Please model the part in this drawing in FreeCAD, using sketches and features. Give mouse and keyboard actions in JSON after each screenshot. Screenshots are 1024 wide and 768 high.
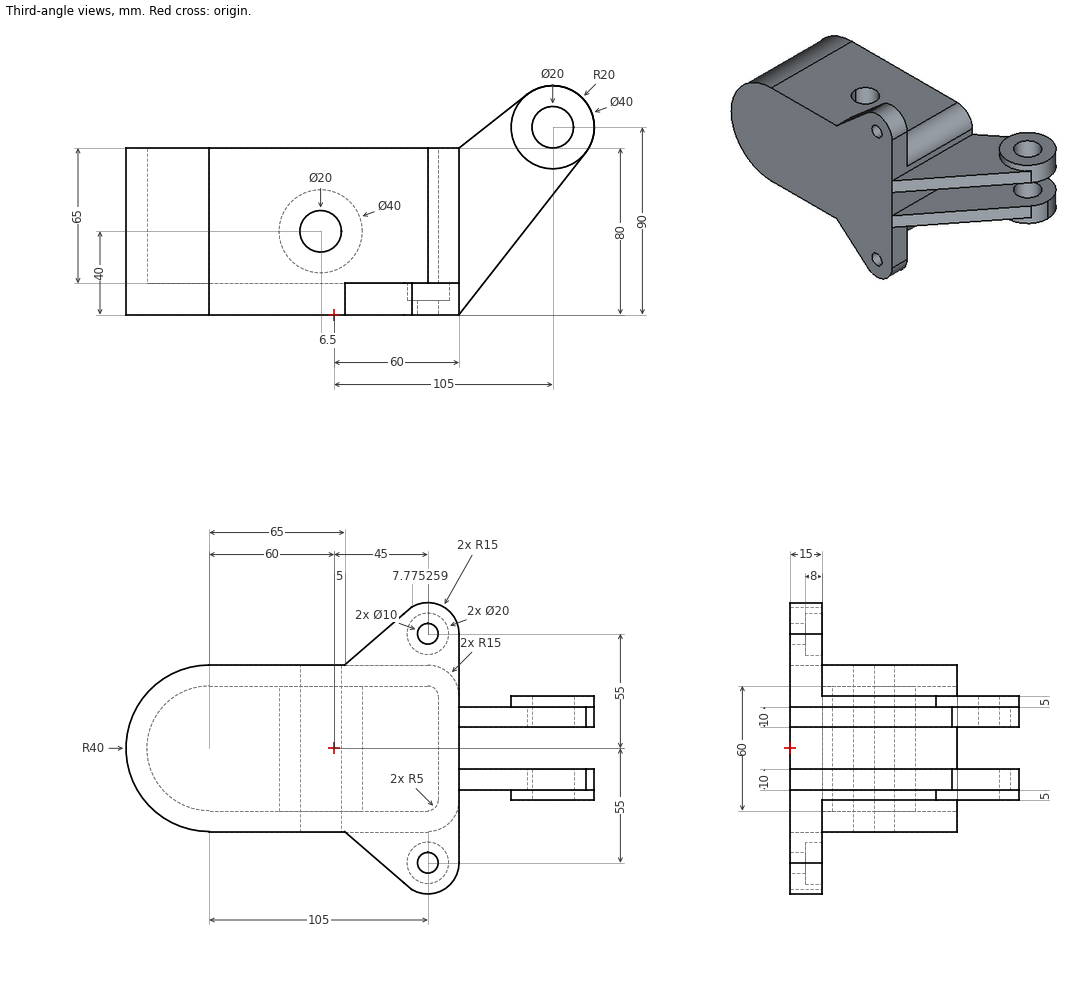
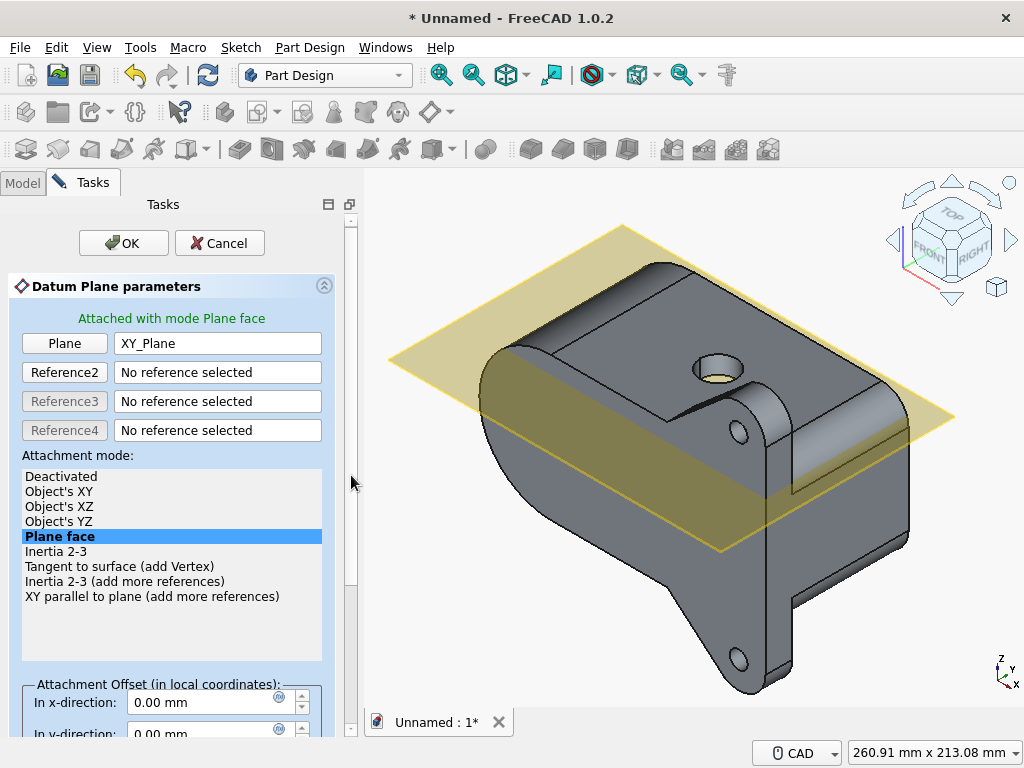
{"action": "left_click", "coordinate": [124, 243]}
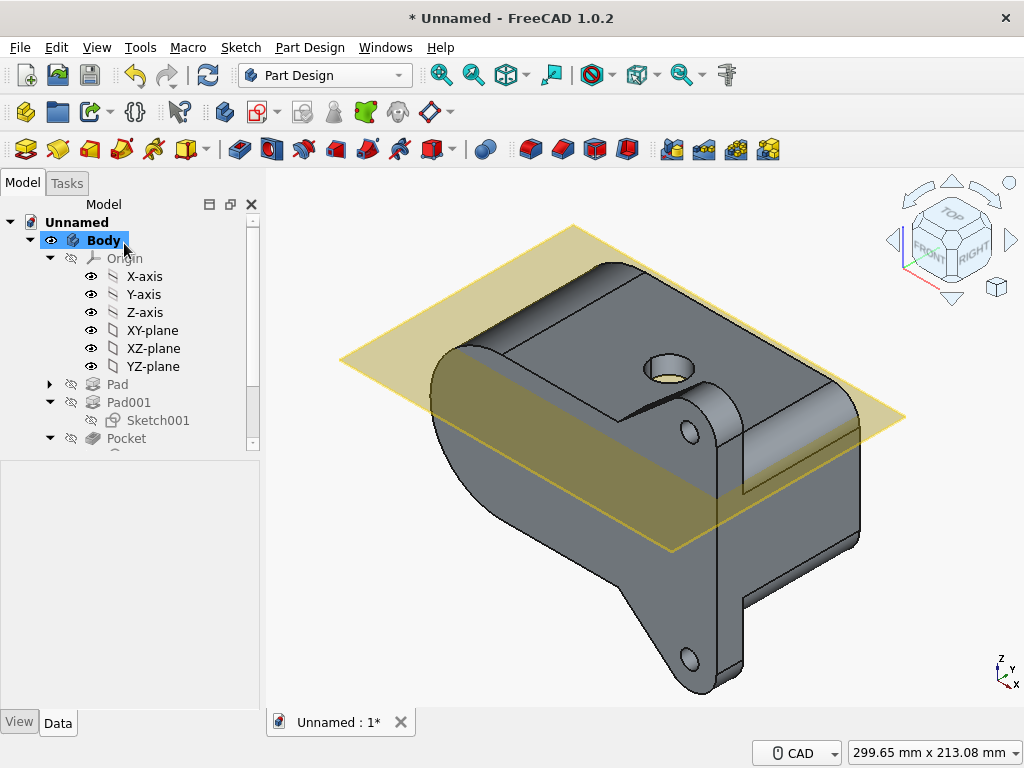
{"action": "scroll", "coordinate": [100, 326], "scroll_direction": "down", "scroll_amount": 3}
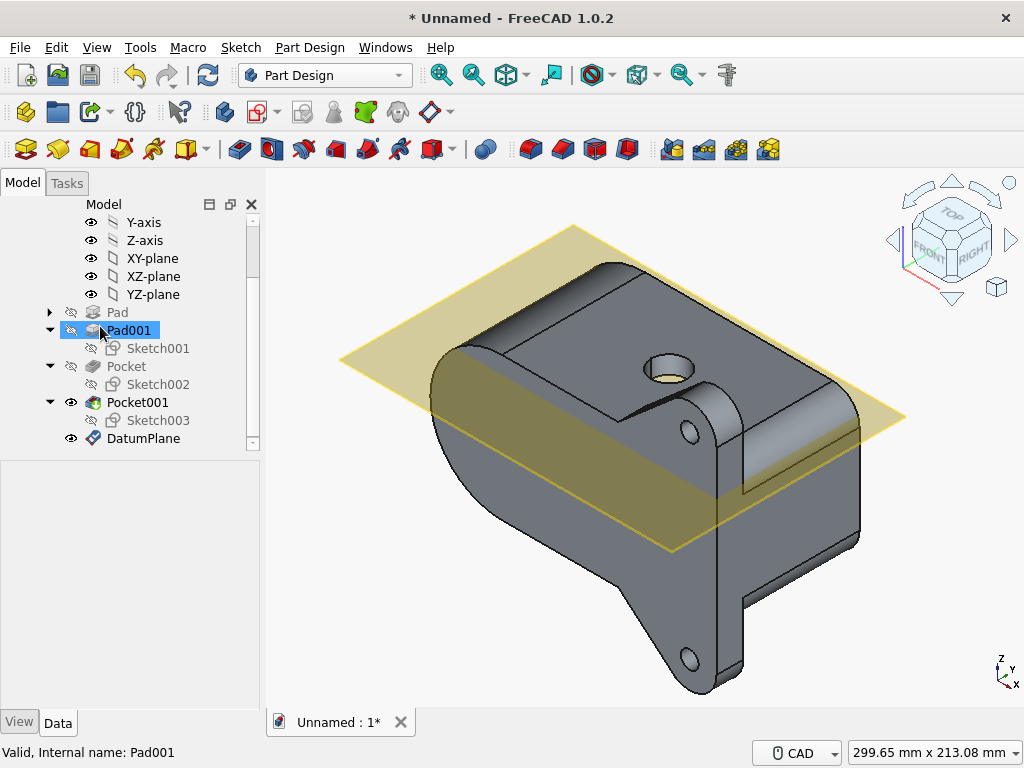
{"action": "left_click", "coordinate": [116, 438]}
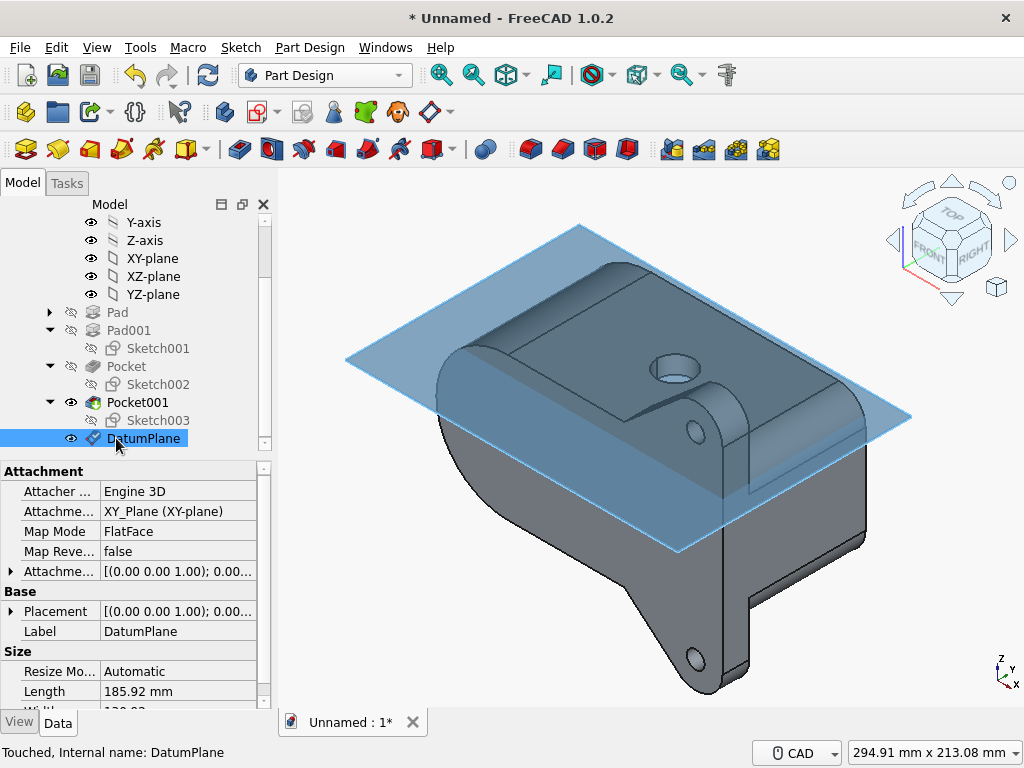
{"action": "left_click", "coordinate": [258, 112]}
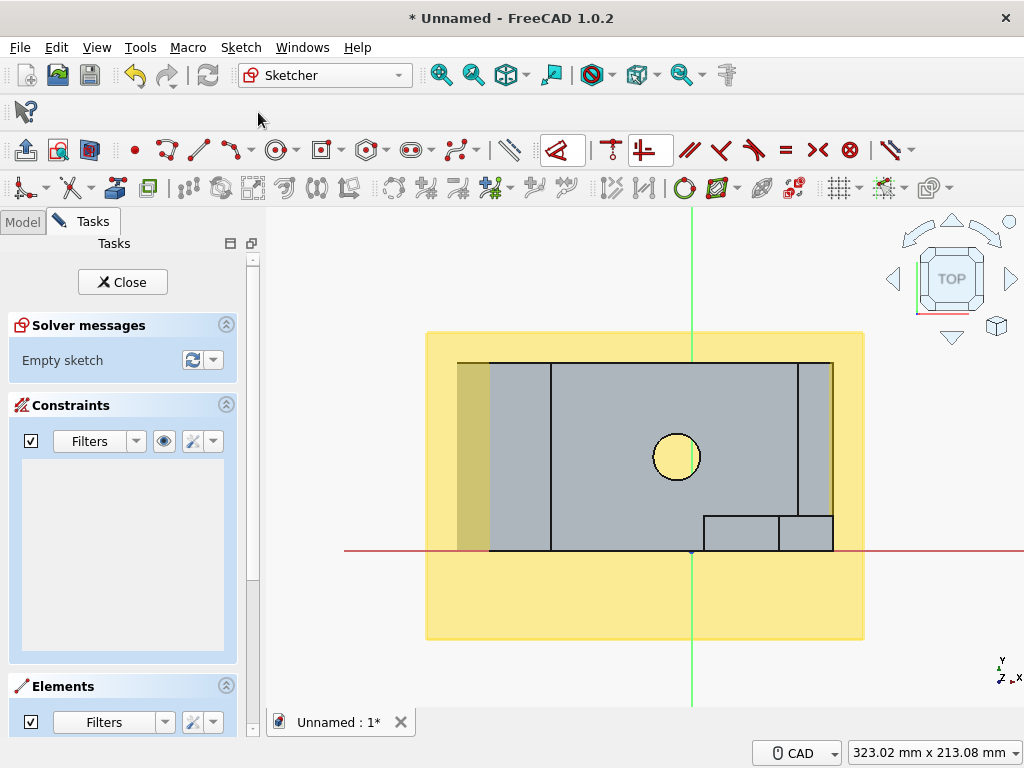
{"action": "left_click", "coordinate": [90, 150]}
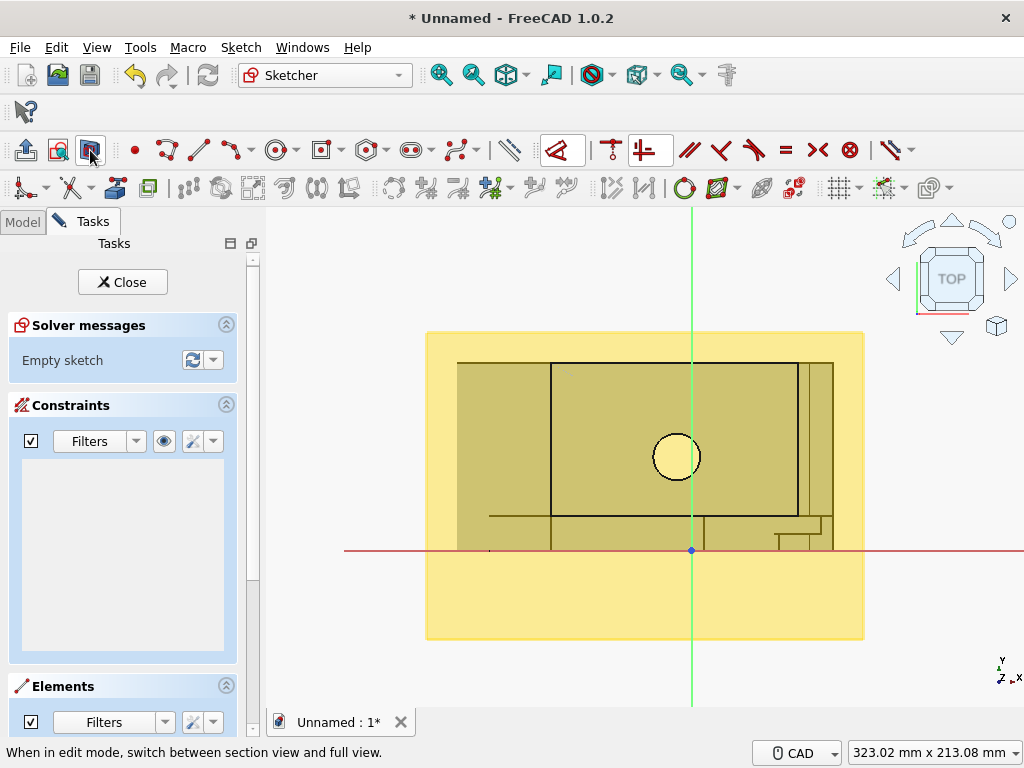
{"action": "scroll", "coordinate": [758, 500], "scroll_direction": "up", "scroll_amount": 4}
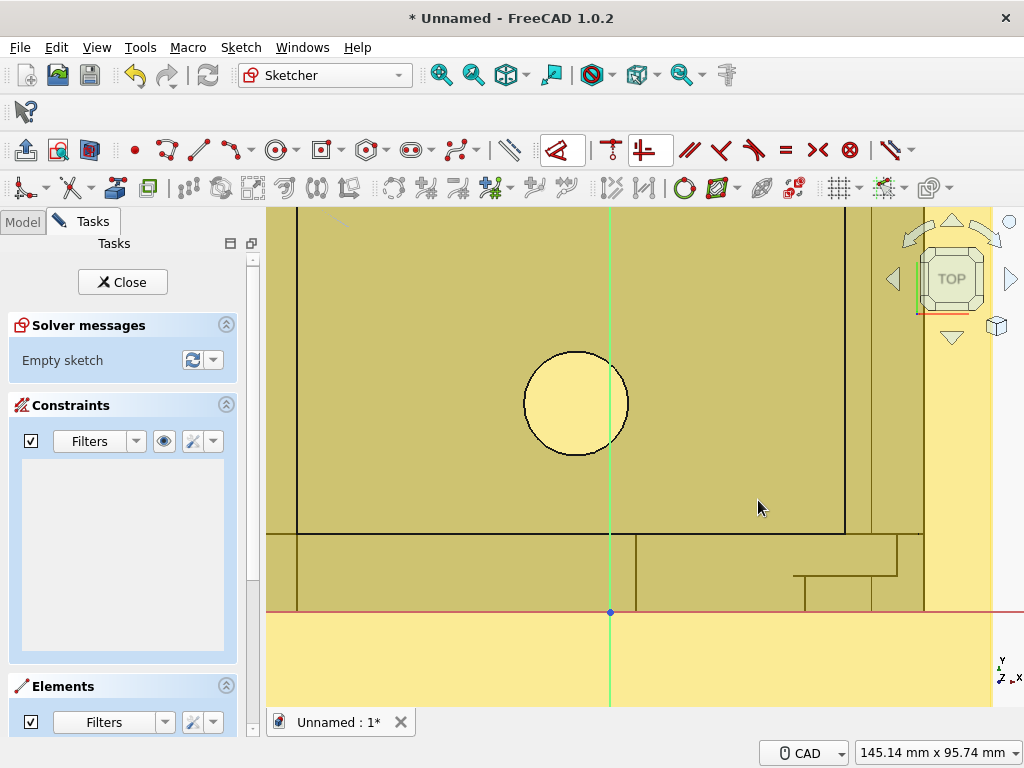
{"action": "left_click", "coordinate": [276, 150]}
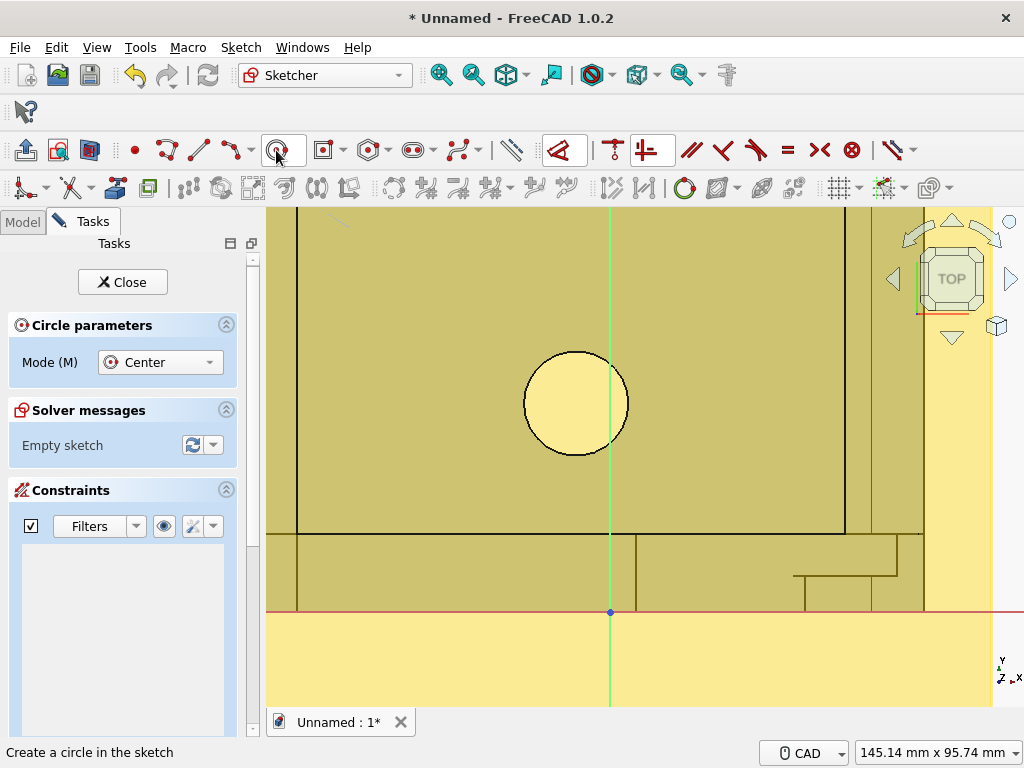
{"action": "left_click", "coordinate": [576, 404]}
{"action": "left_click", "coordinate": [650, 330]}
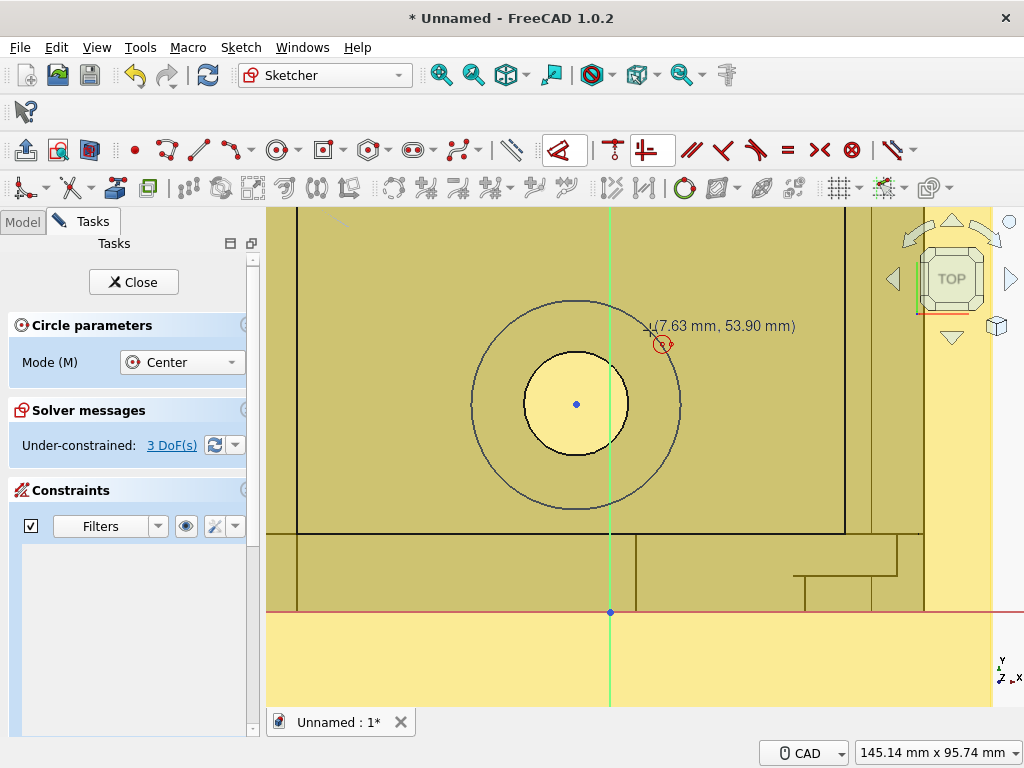
{"action": "left_click", "coordinate": [576, 405]}
{"action": "left_click", "coordinate": [539, 367]}
{"action": "key", "text": "Escape"}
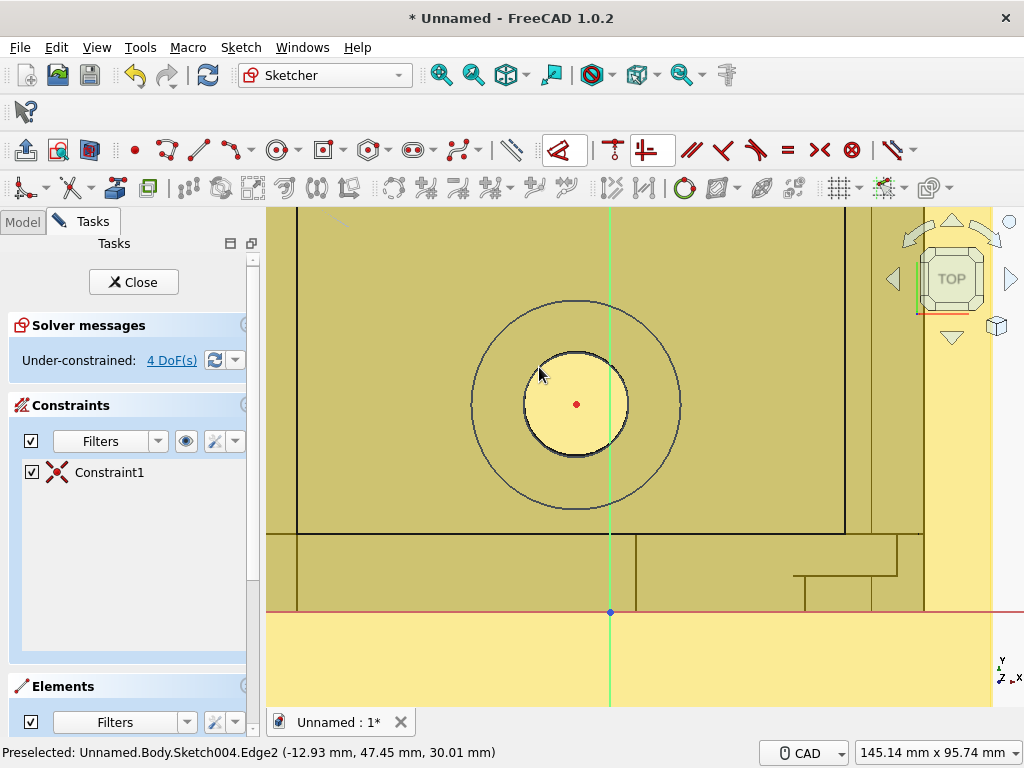
{"action": "left_click", "coordinate": [650, 331]}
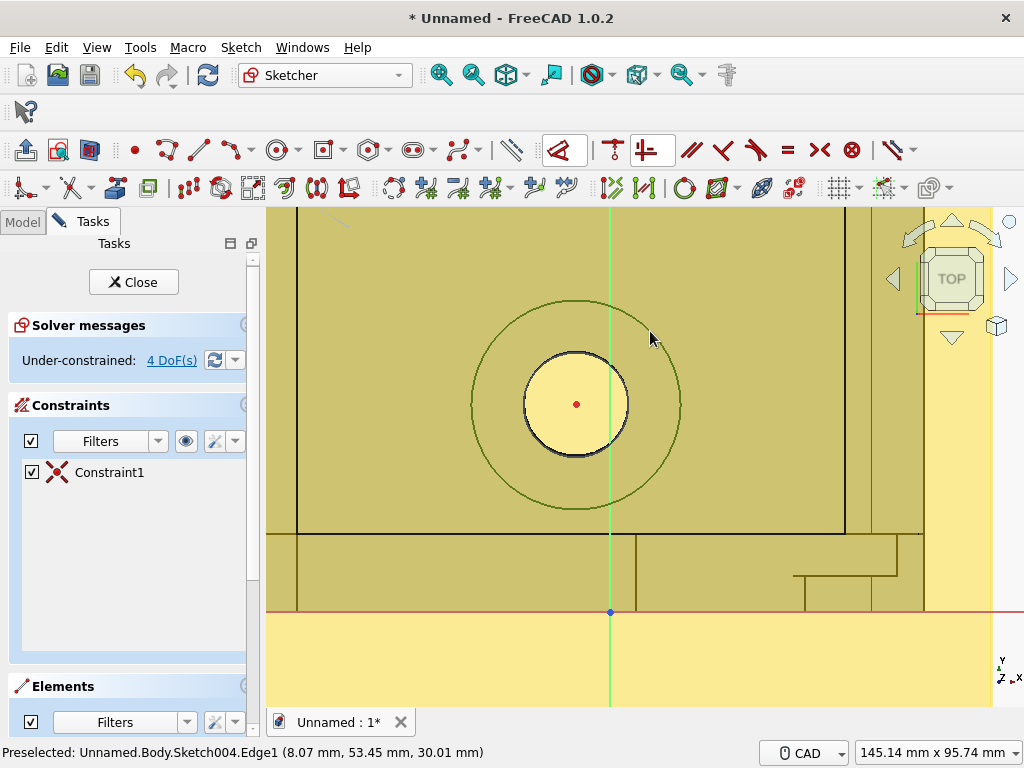
{"action": "left_click", "coordinate": [582, 150]}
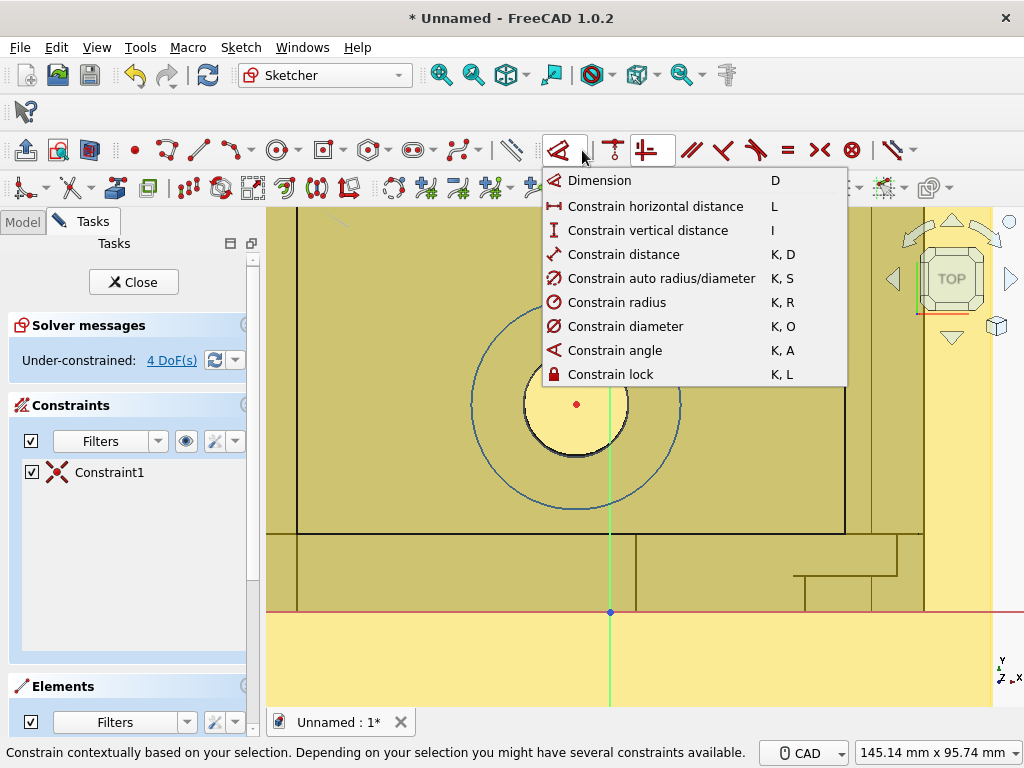
{"action": "left_click", "coordinate": [695, 326]}